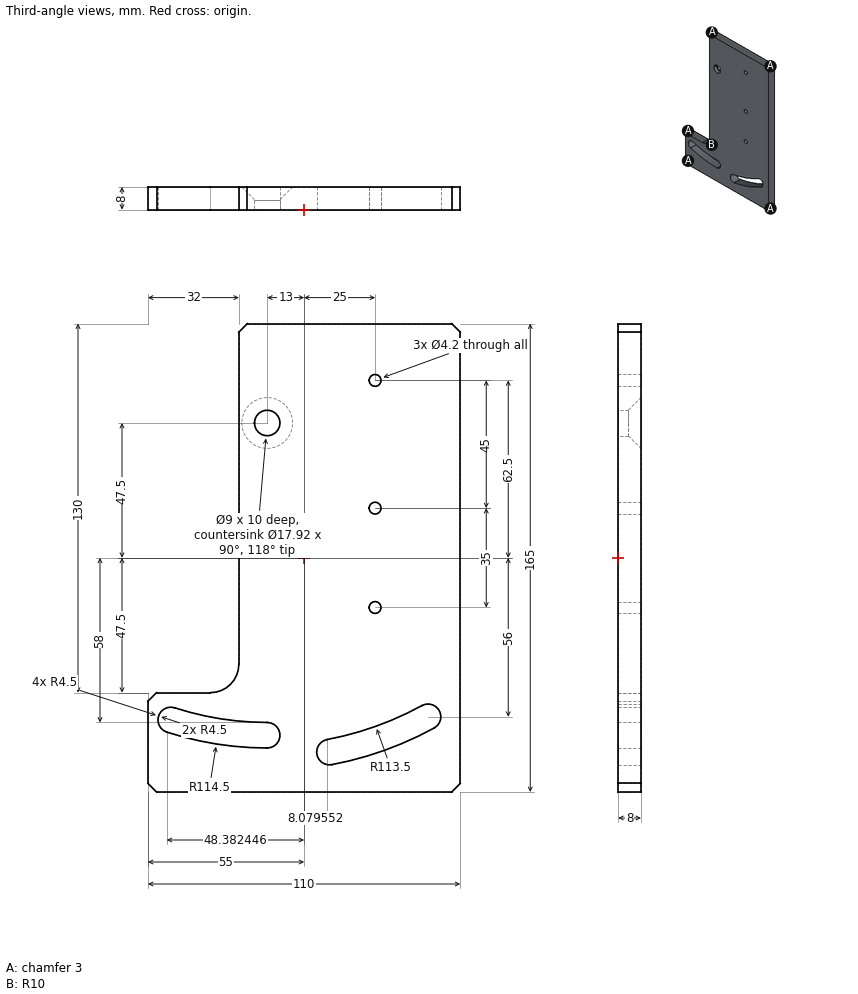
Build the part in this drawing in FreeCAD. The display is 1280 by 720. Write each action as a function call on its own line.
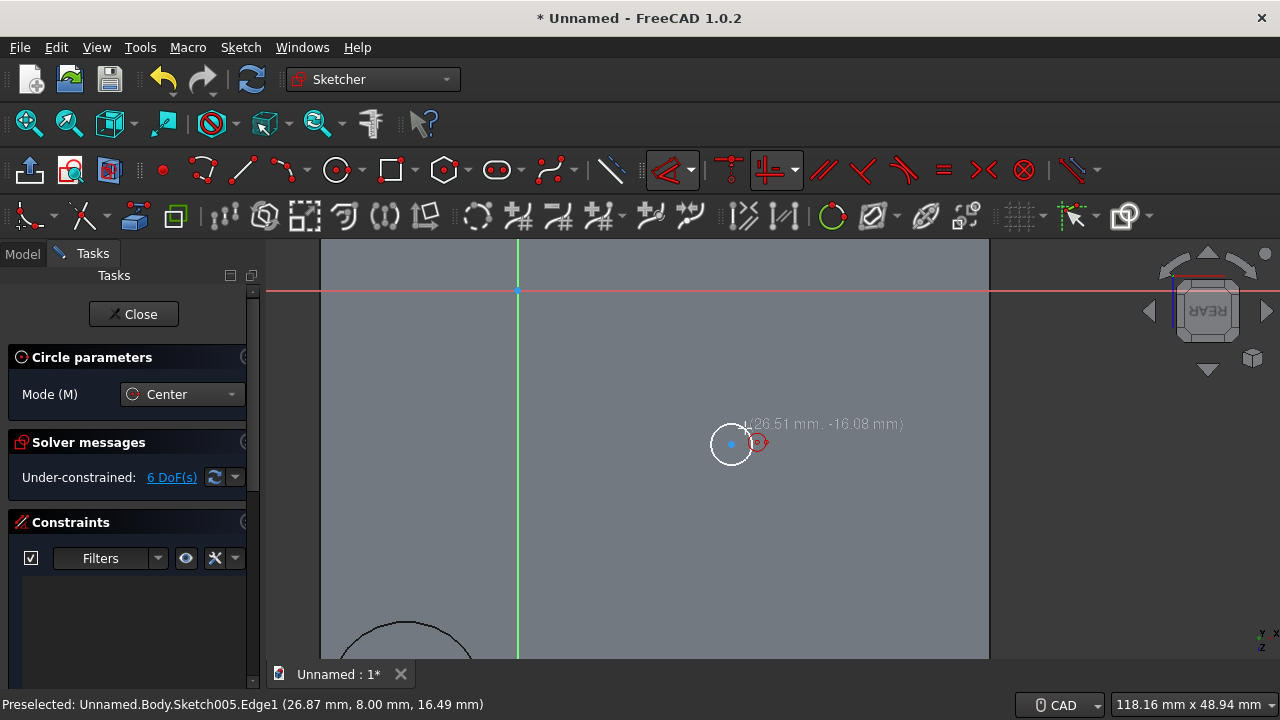
scroll(746, 429, down, 5)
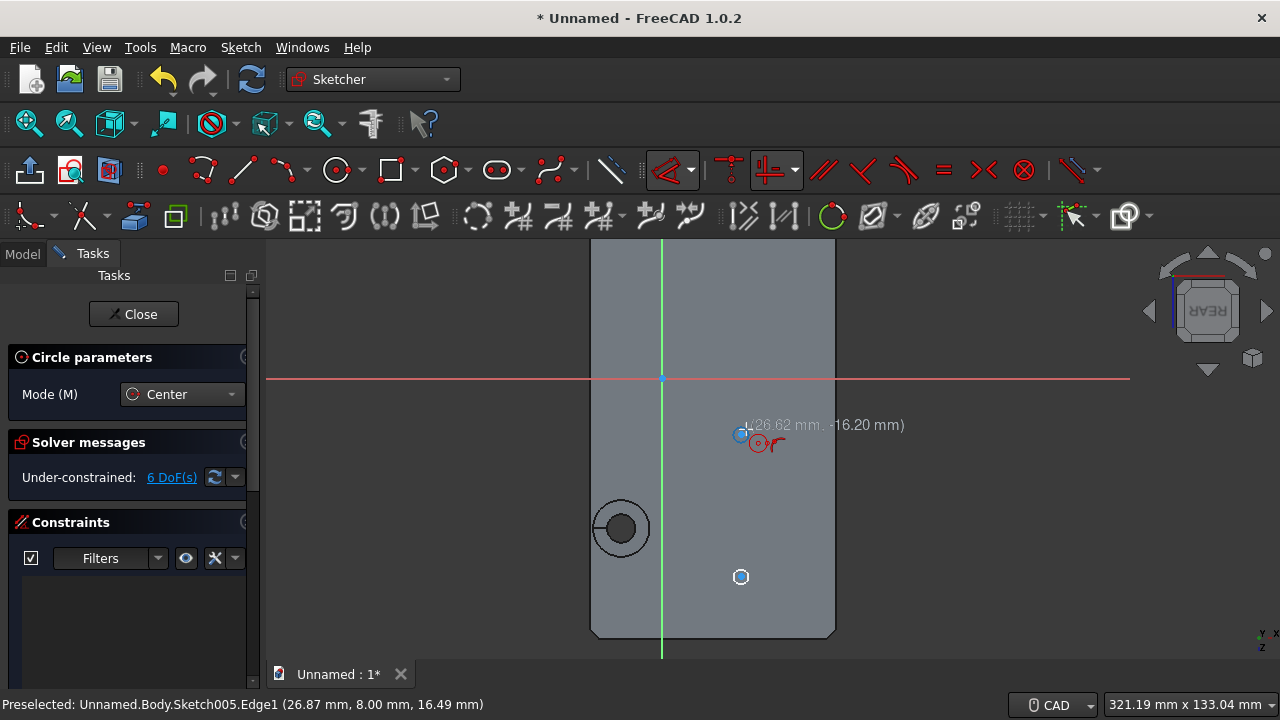
scroll(741, 323, up, 7)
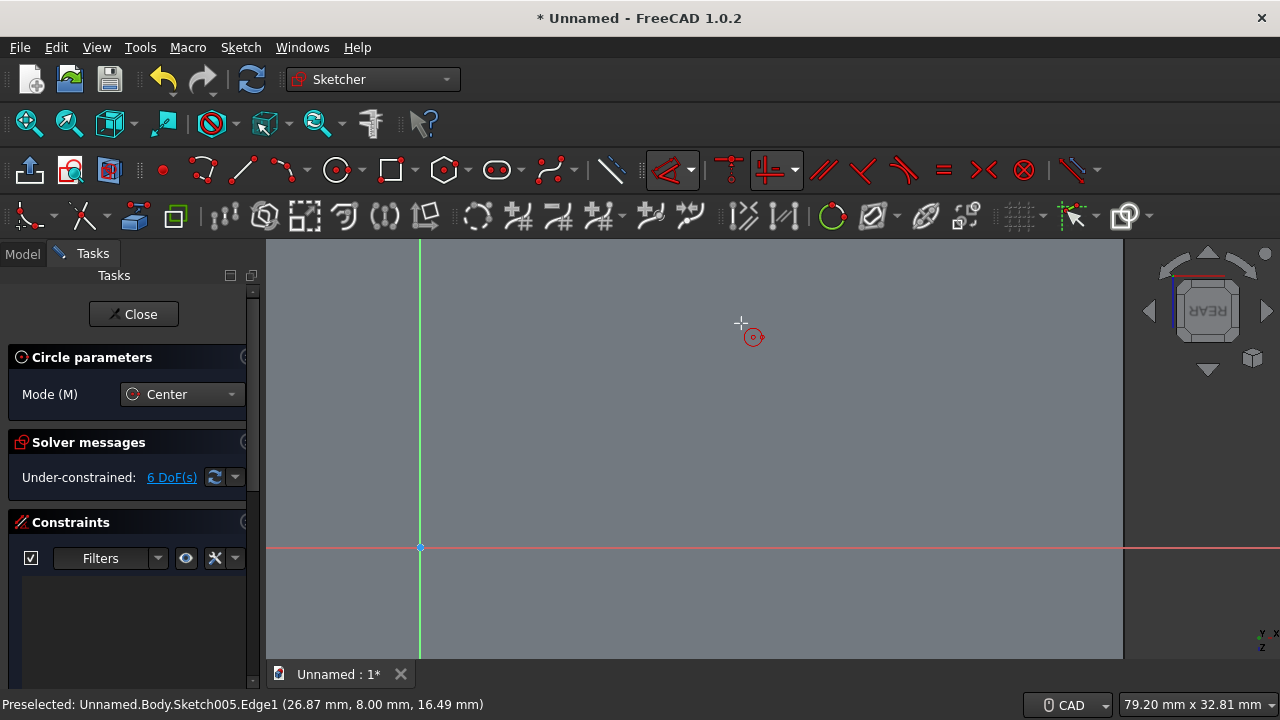
scroll(741, 322, down, 7)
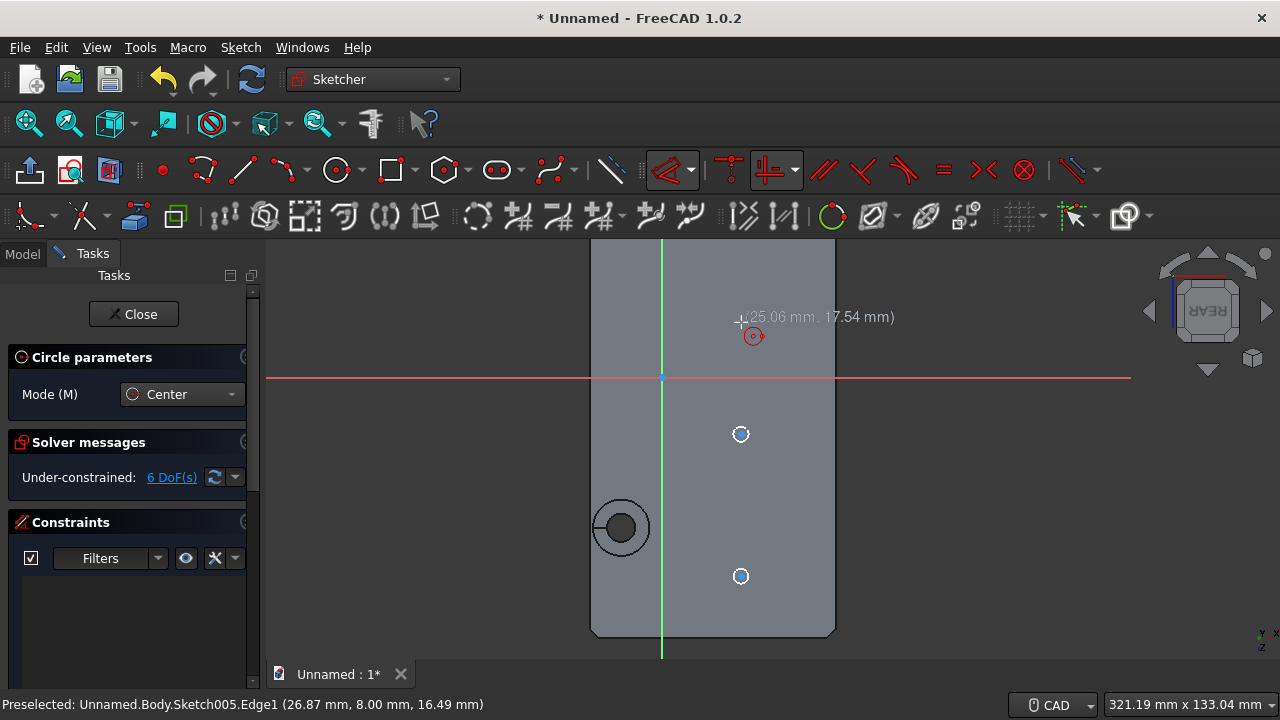
click(741, 323)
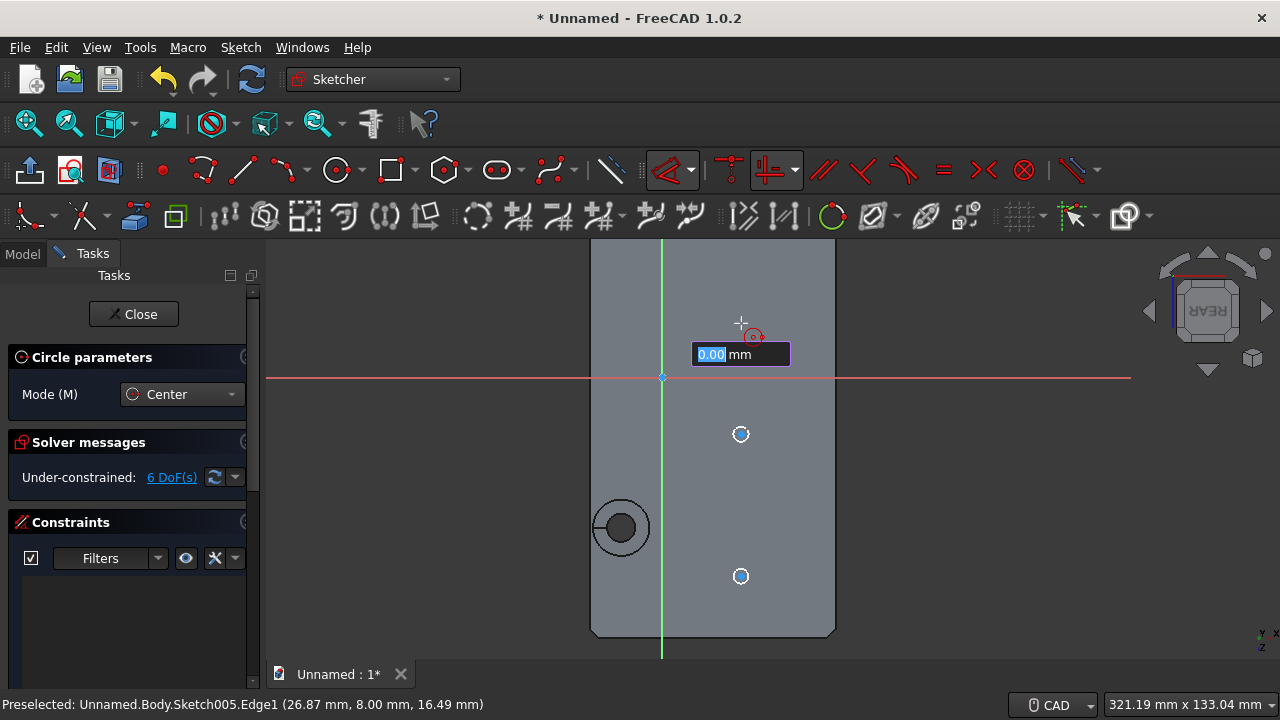
scroll(746, 318, up, 5)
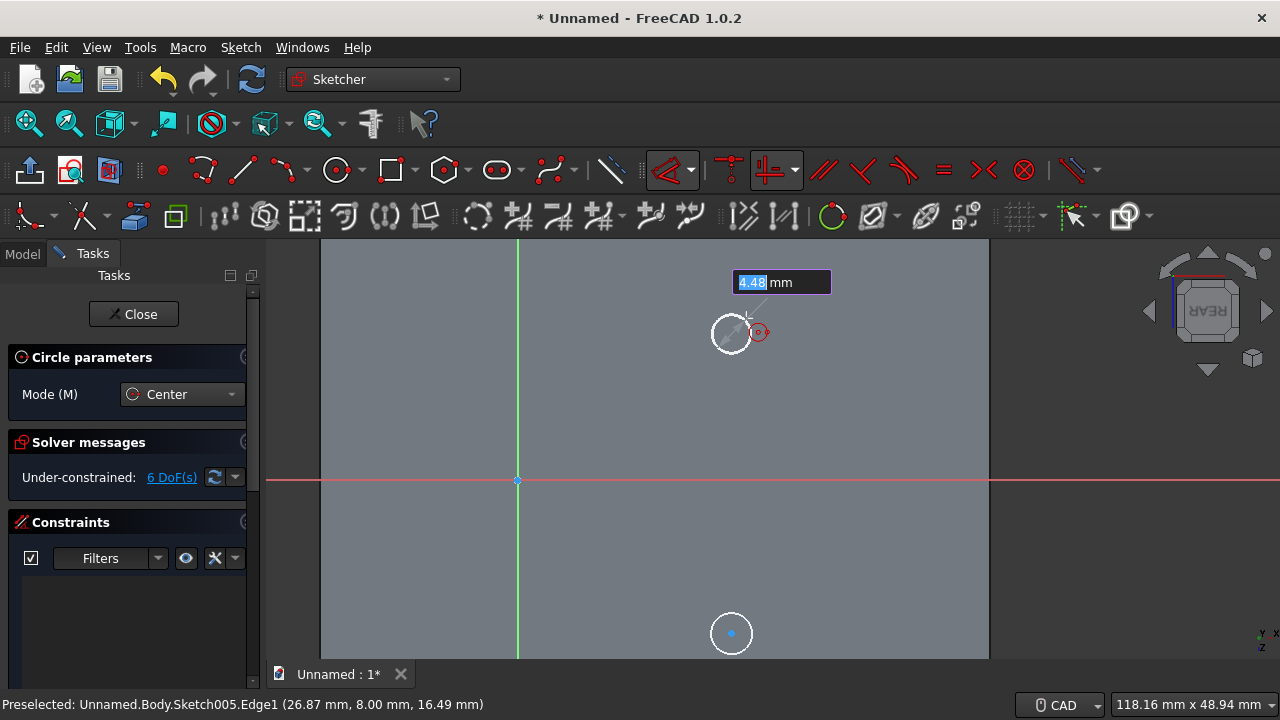
click(745, 317)
key(Escape)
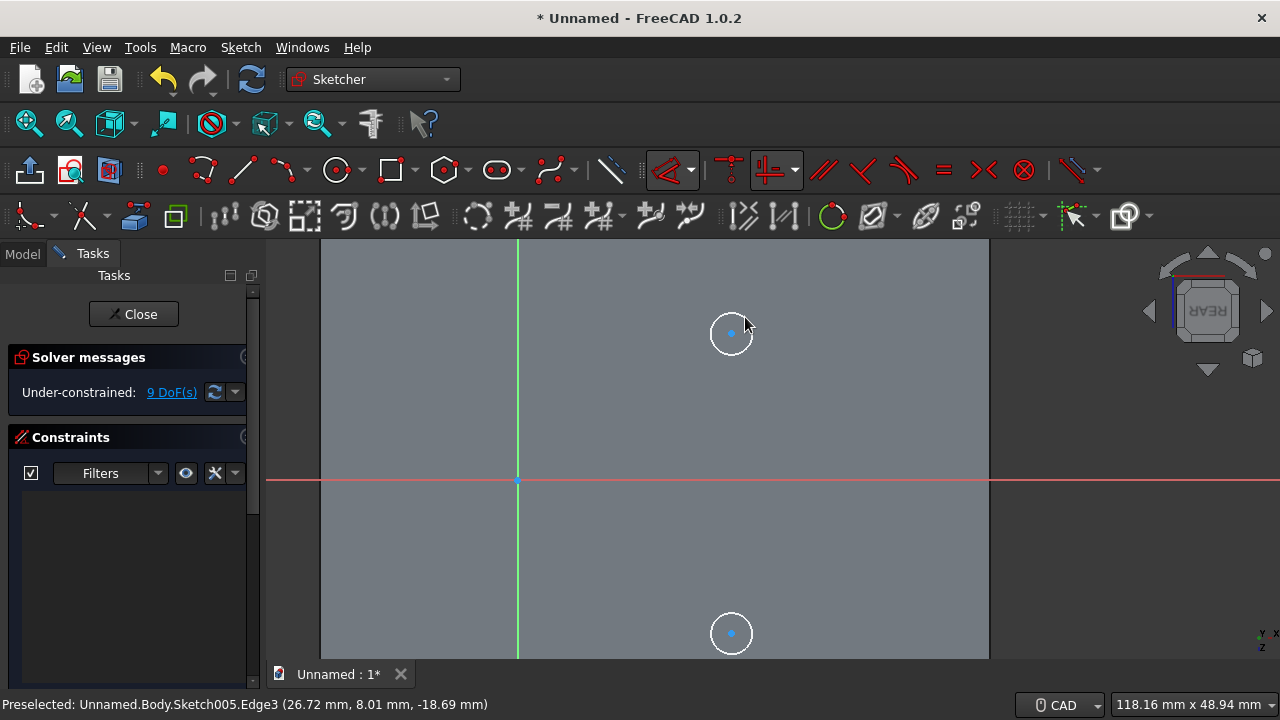
scroll(746, 319, down, 5)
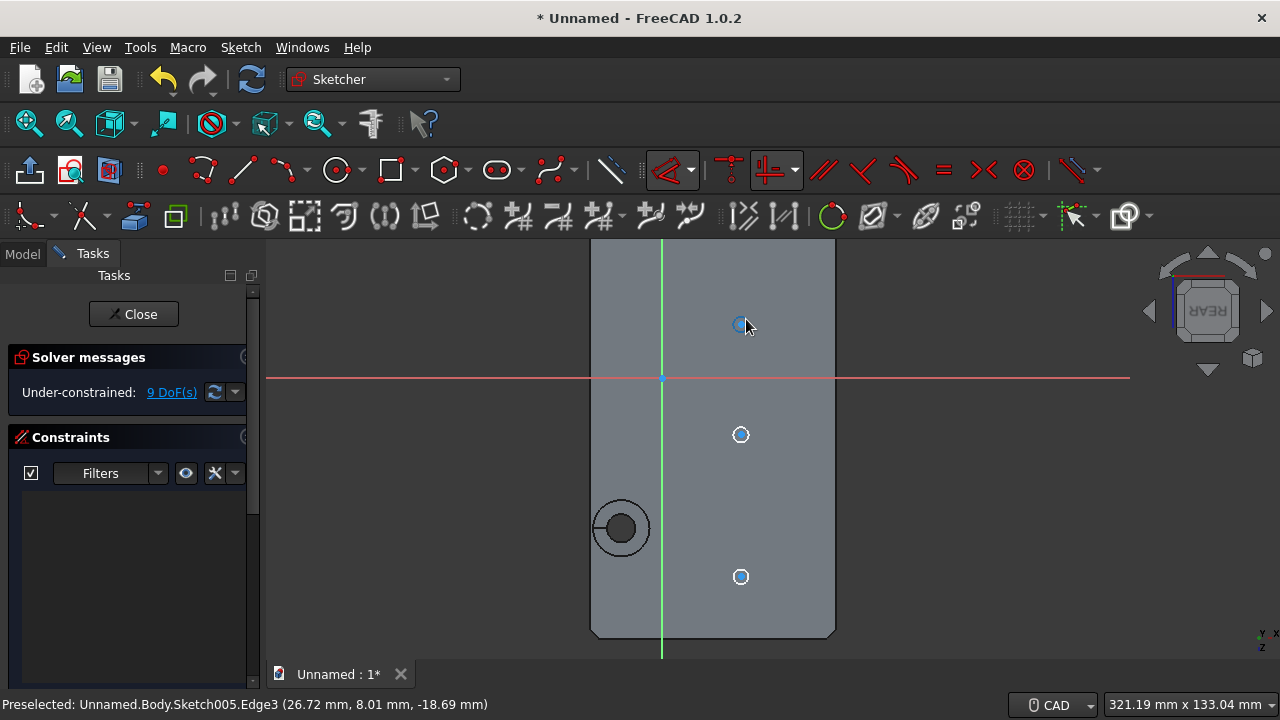
scroll(746, 572, up, 4)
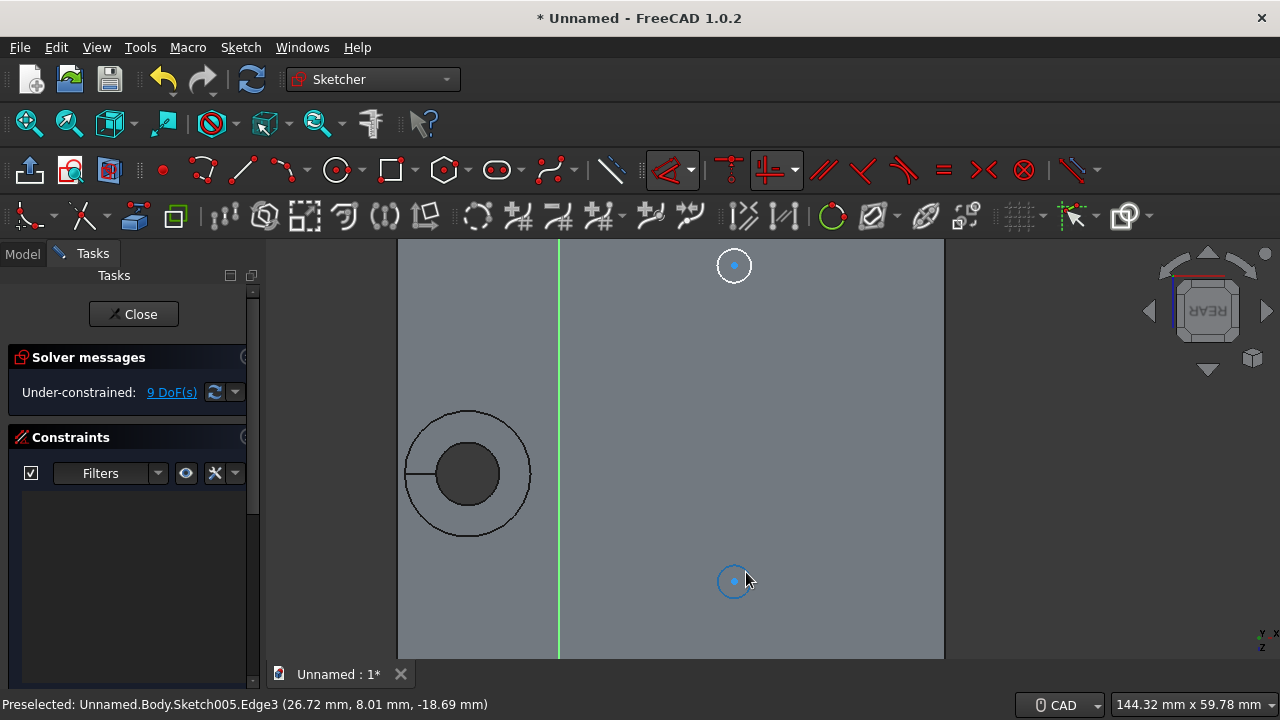
click(746, 570)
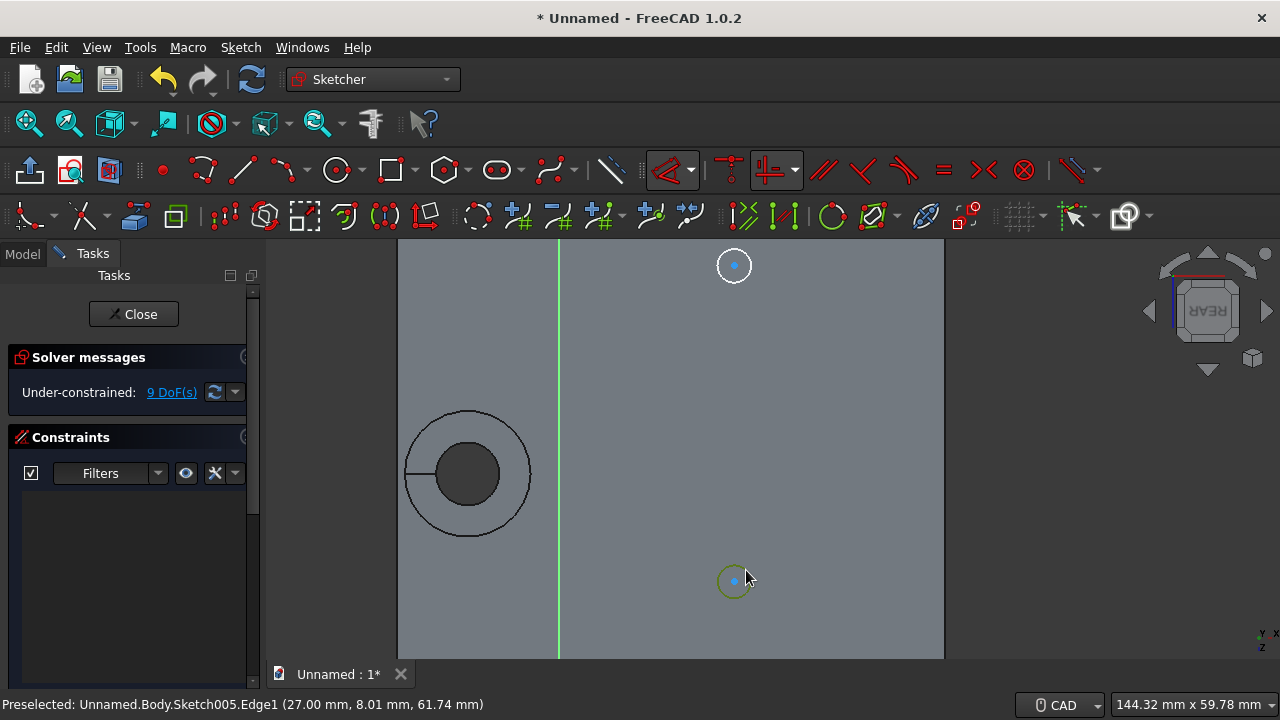
click(722, 278)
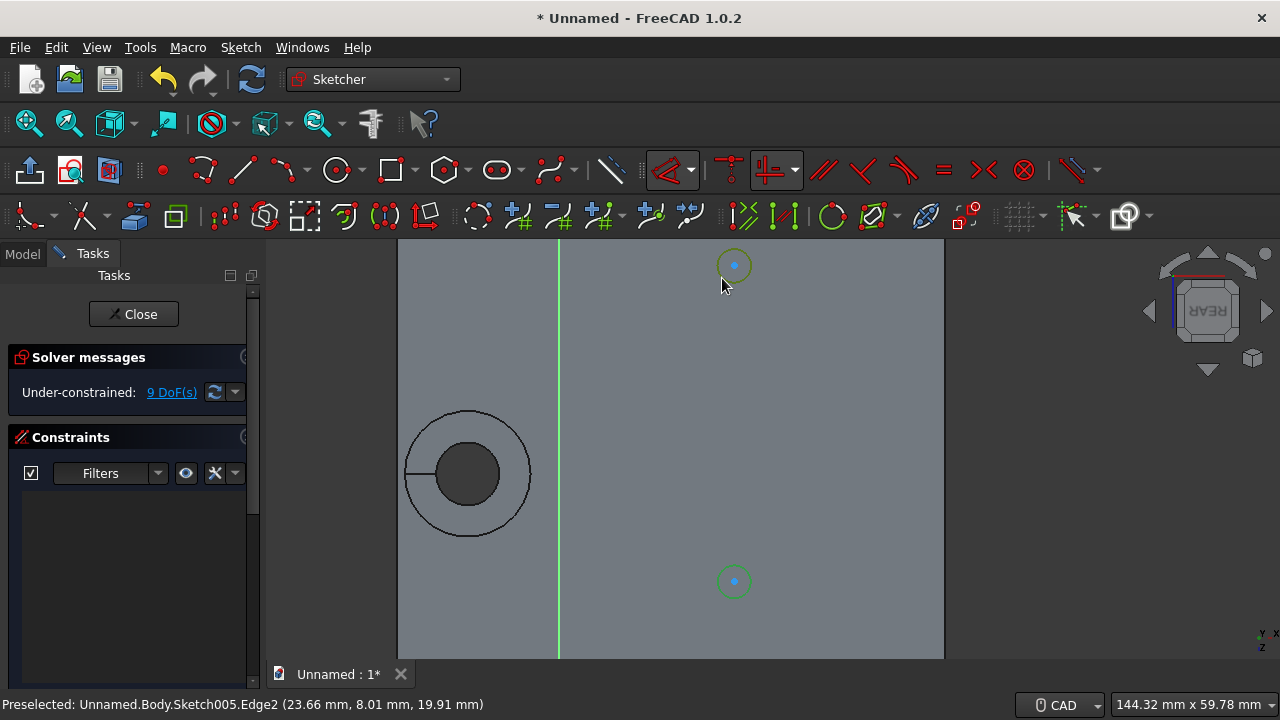
scroll(746, 572, down, 4)